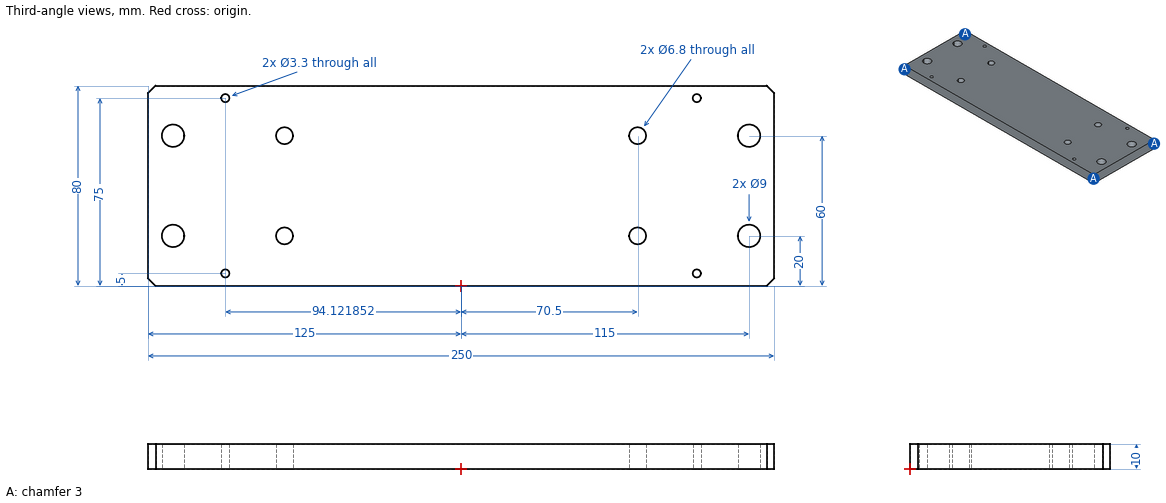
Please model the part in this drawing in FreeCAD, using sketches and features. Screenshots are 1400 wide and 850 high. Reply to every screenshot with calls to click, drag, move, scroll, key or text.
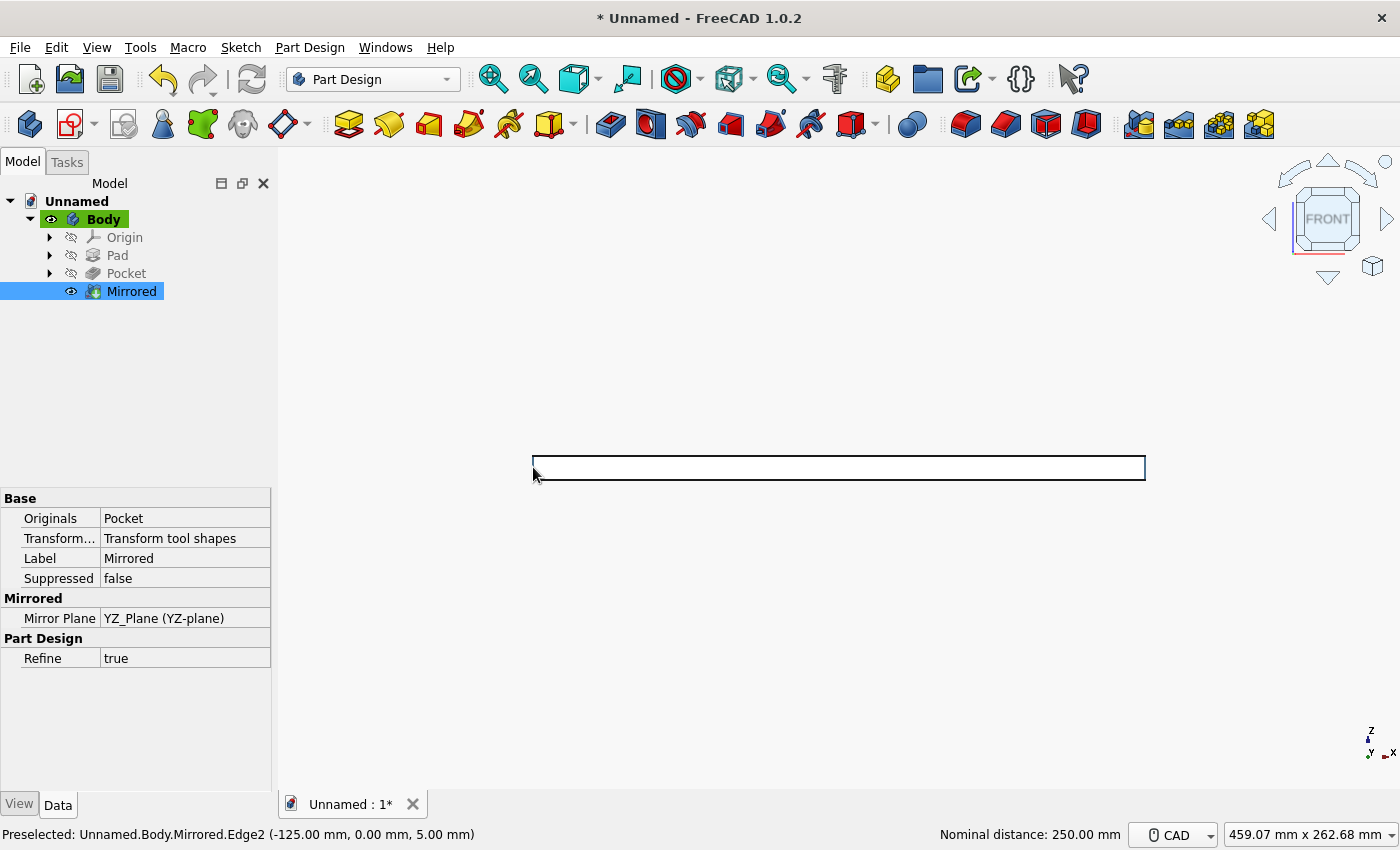
key(3)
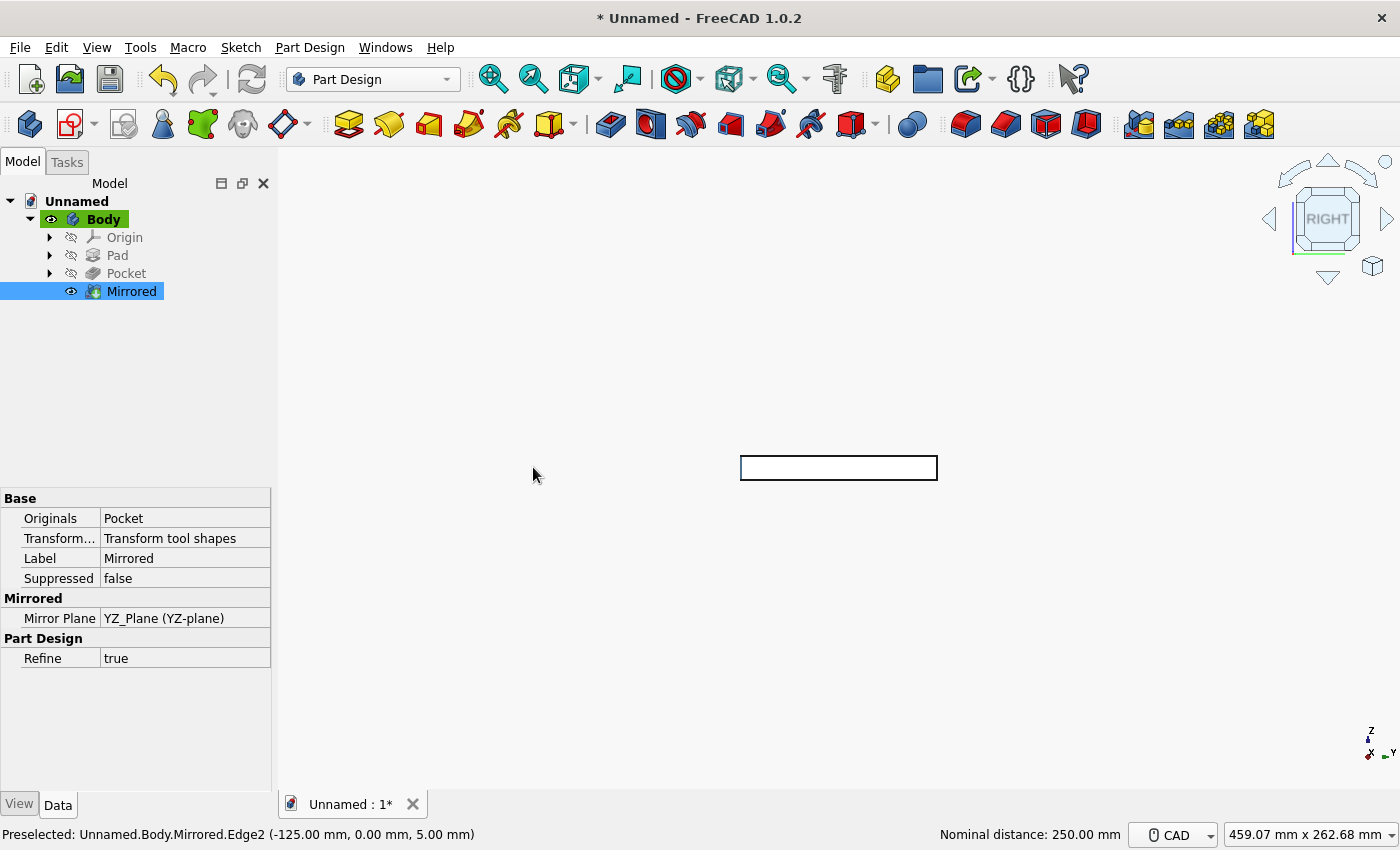
click(494, 80)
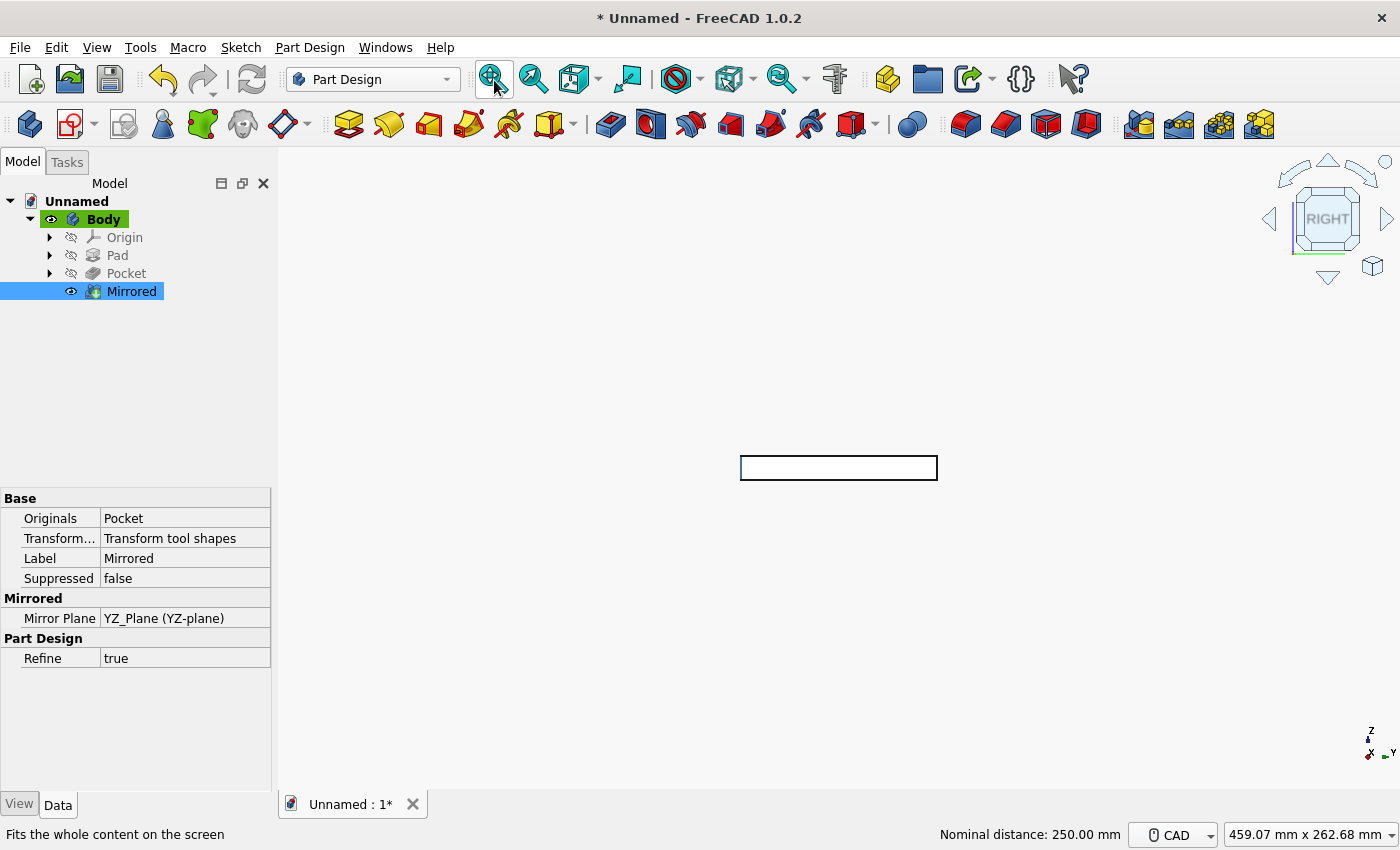
click(937, 467, ctrl)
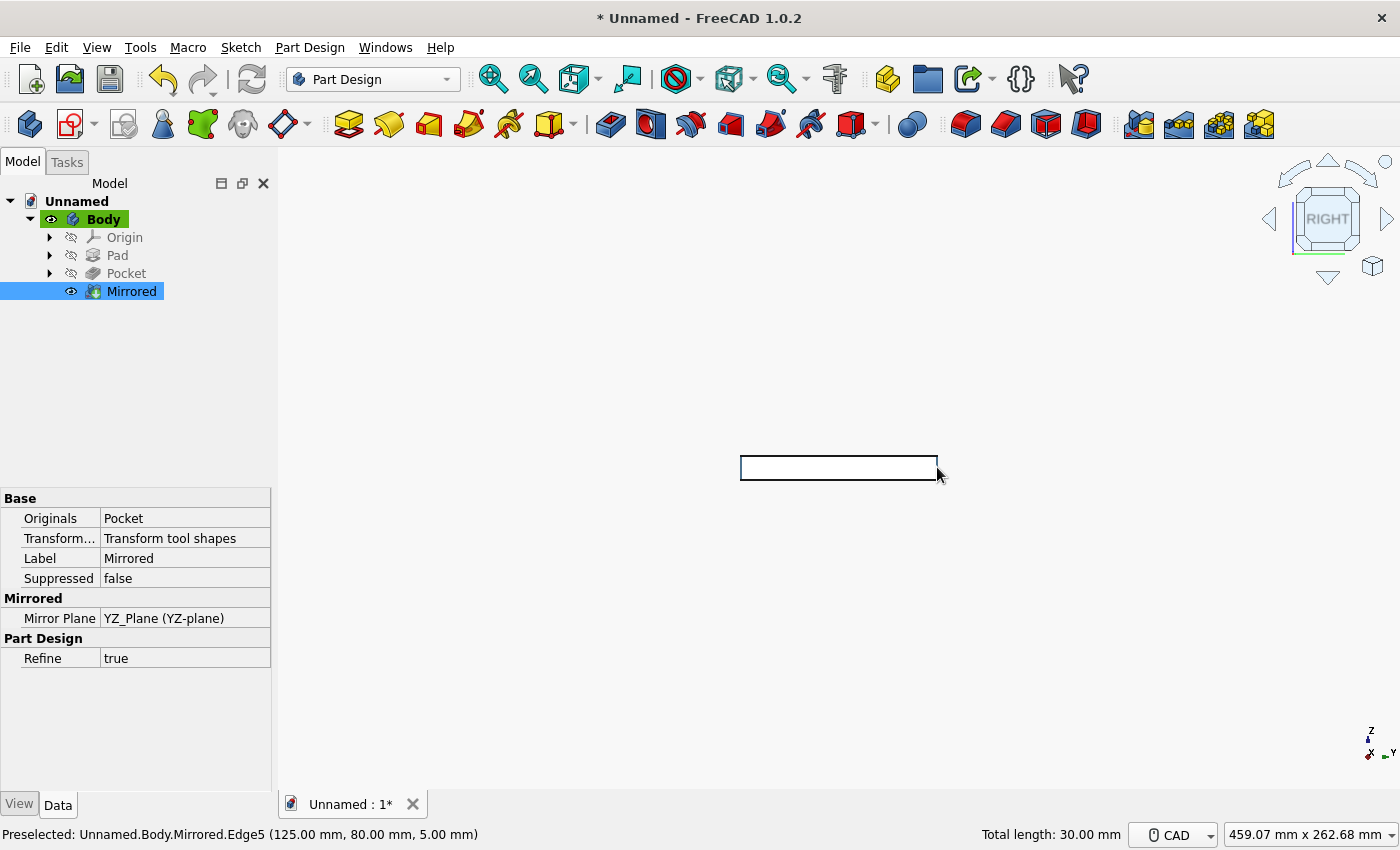
key(5)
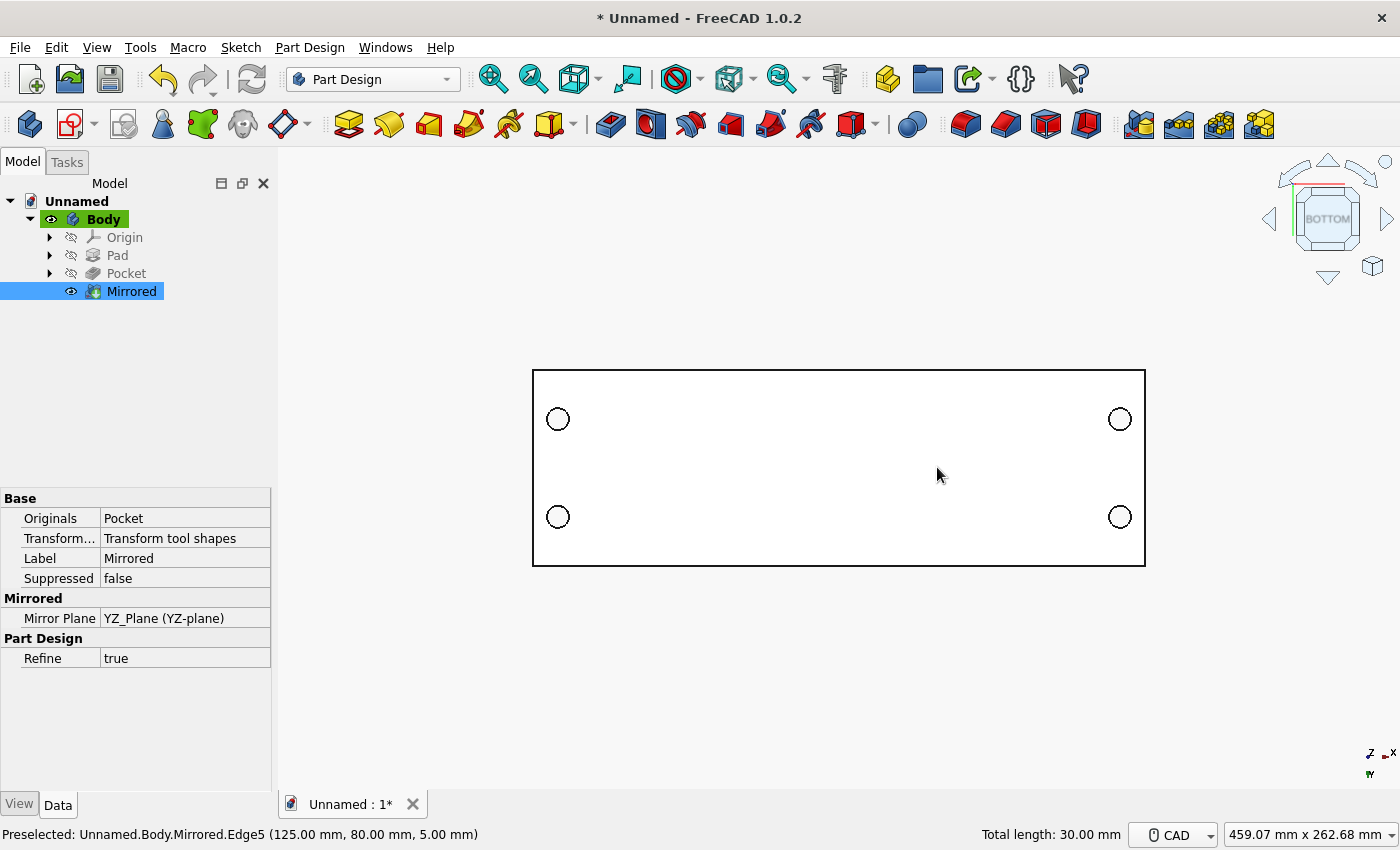
key(4)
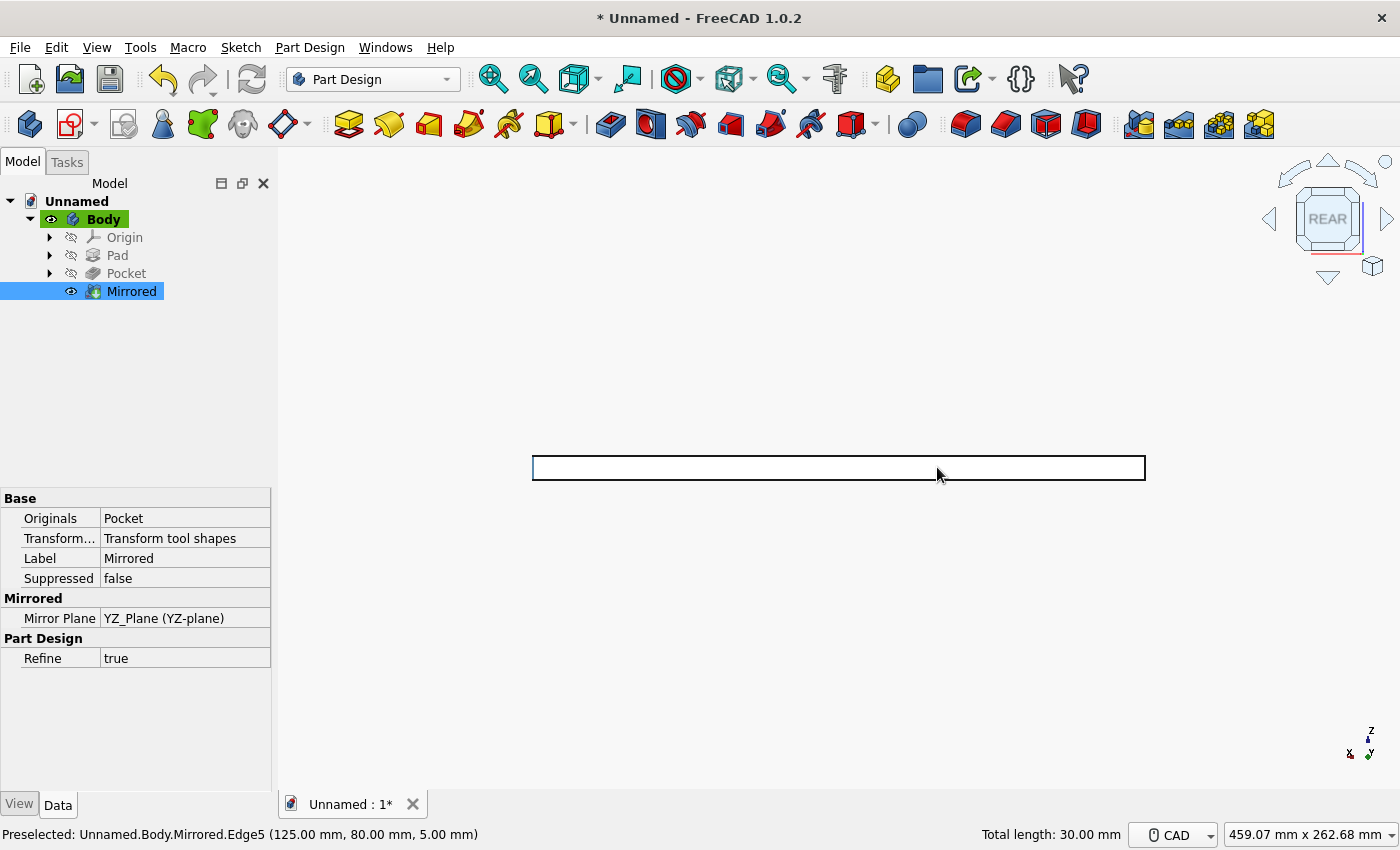
click(1145, 467, ctrl)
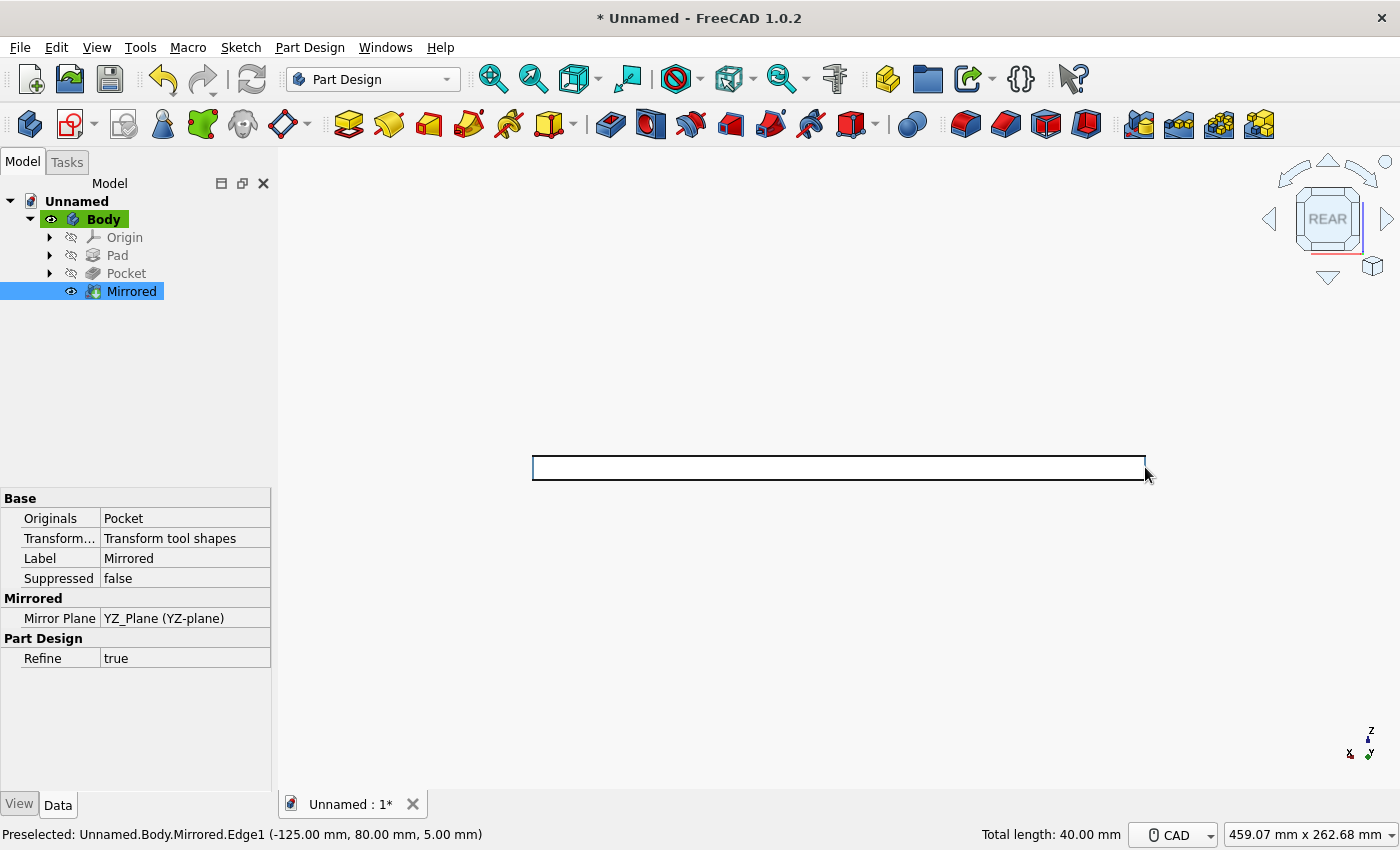
click(1006, 124)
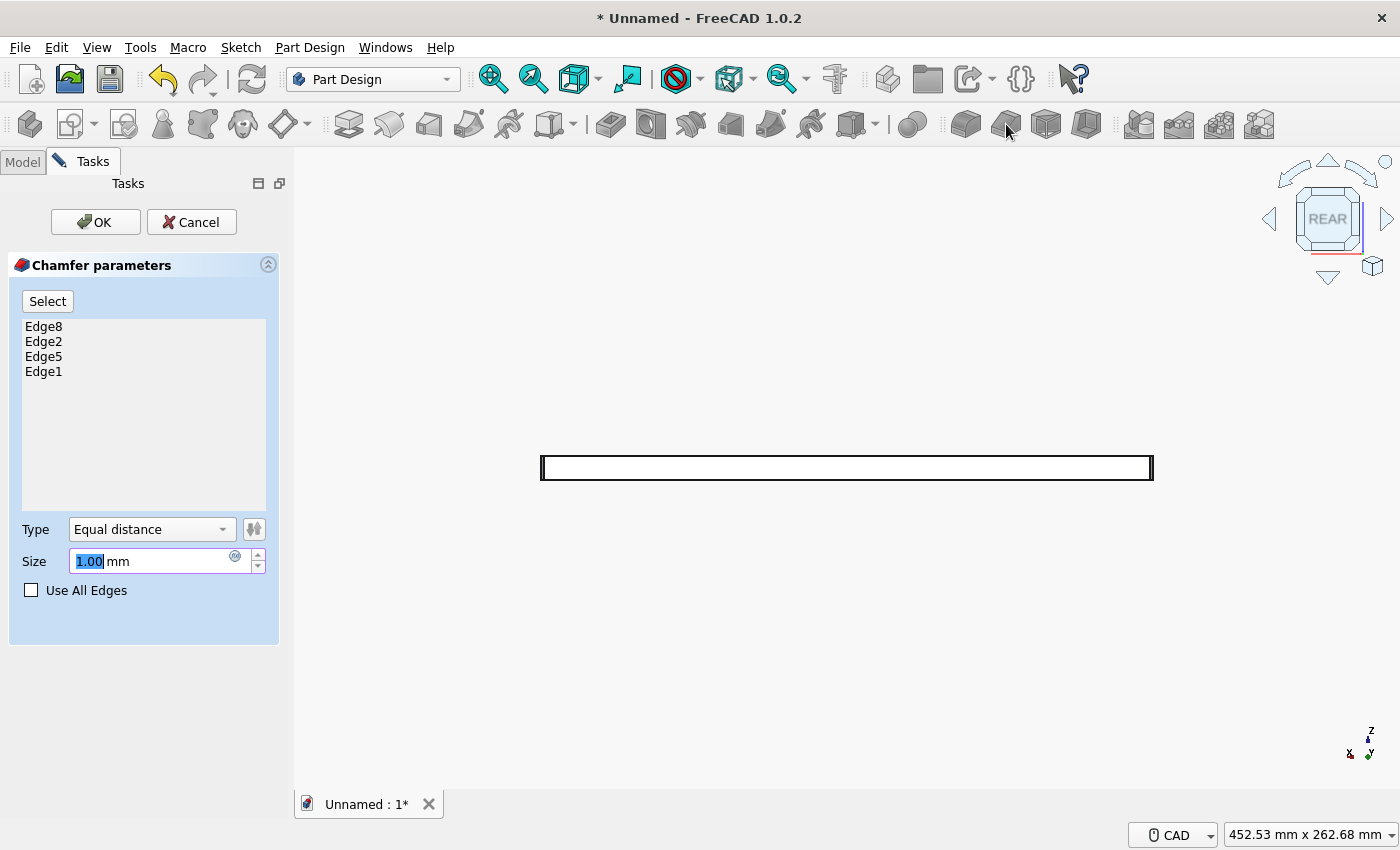
text(3)
key(Tab)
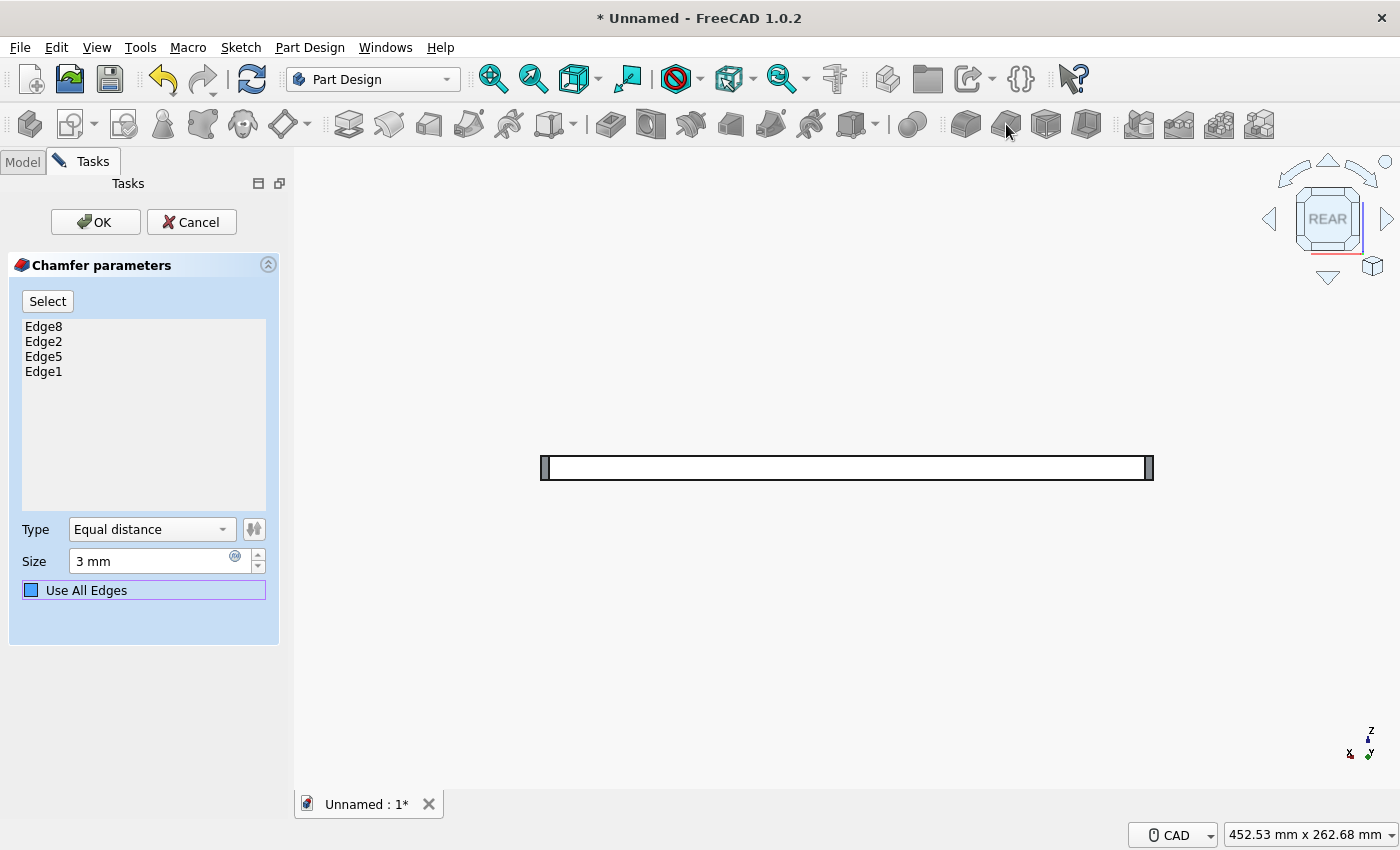
click(96, 222)